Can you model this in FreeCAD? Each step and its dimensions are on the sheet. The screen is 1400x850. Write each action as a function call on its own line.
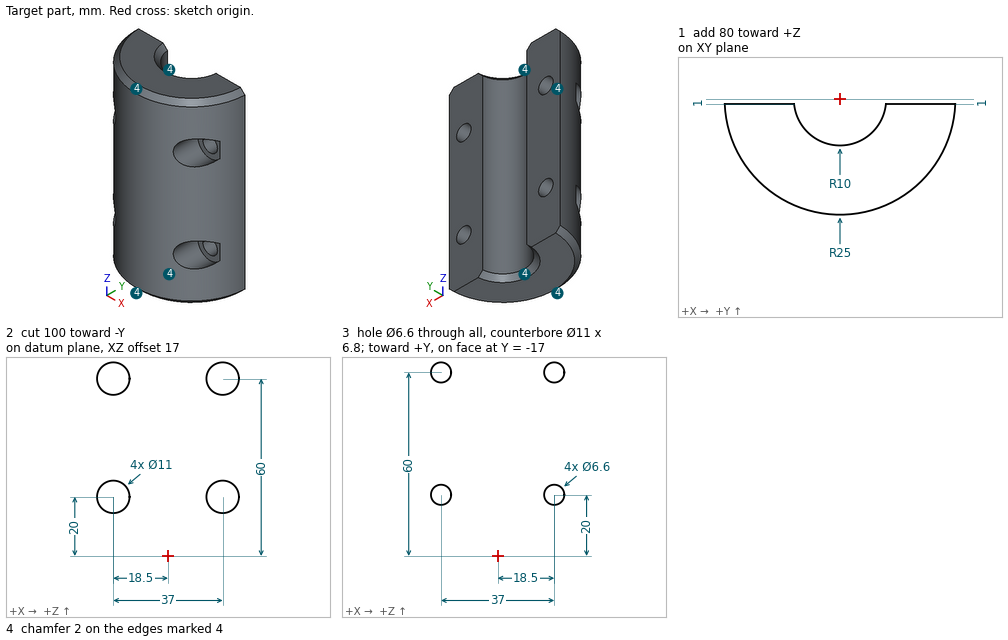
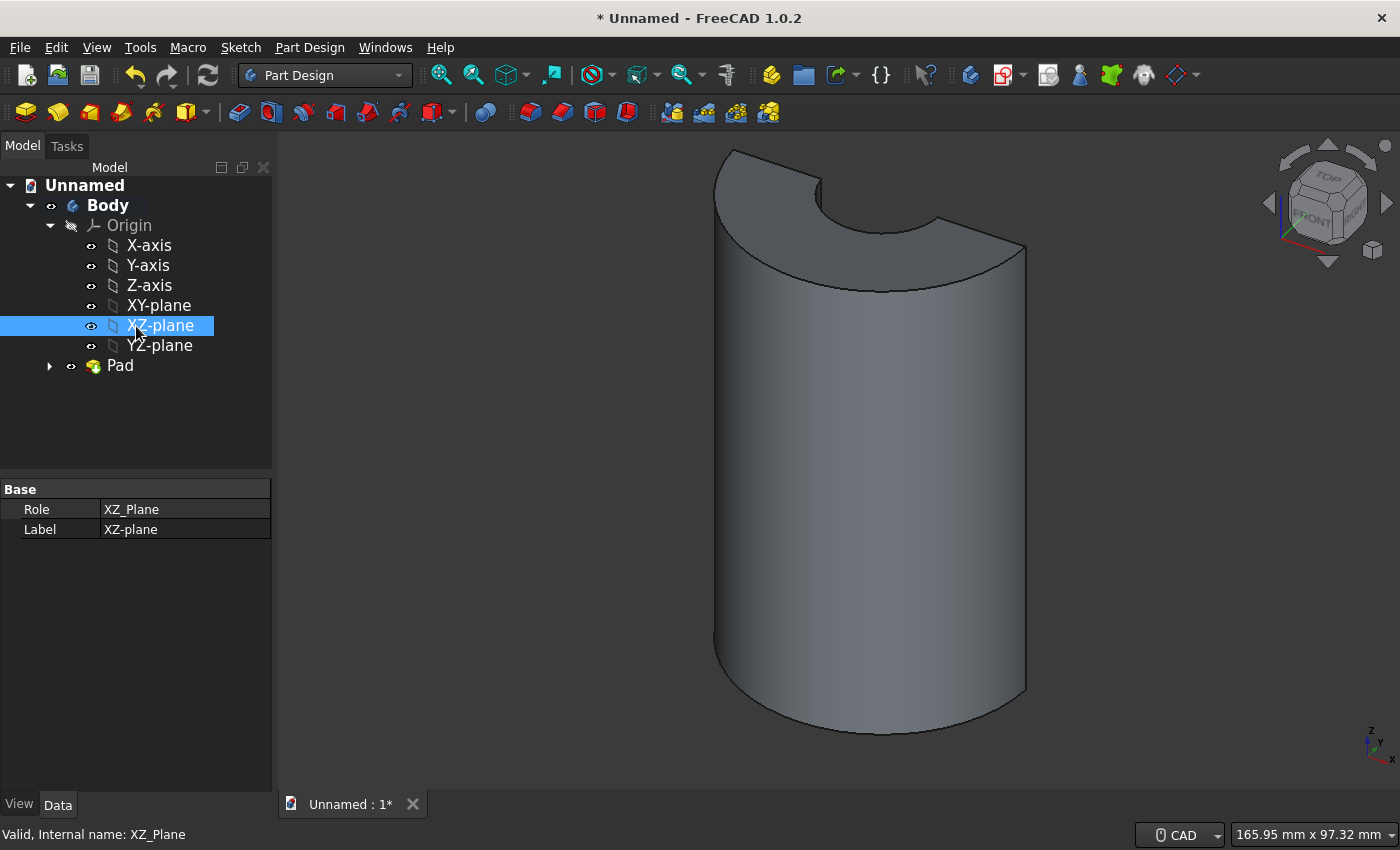
click(1176, 76)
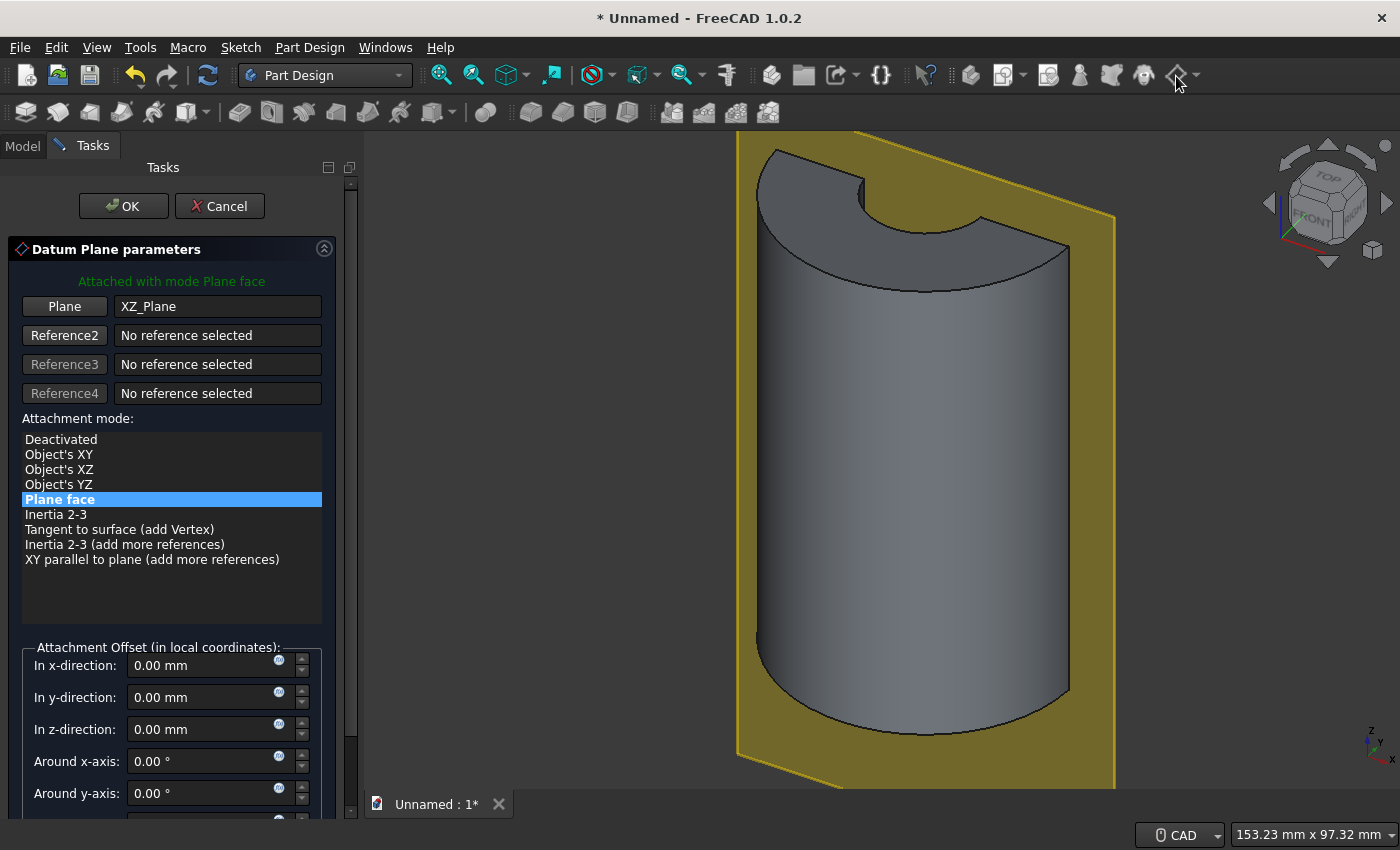
triple_click(210, 729)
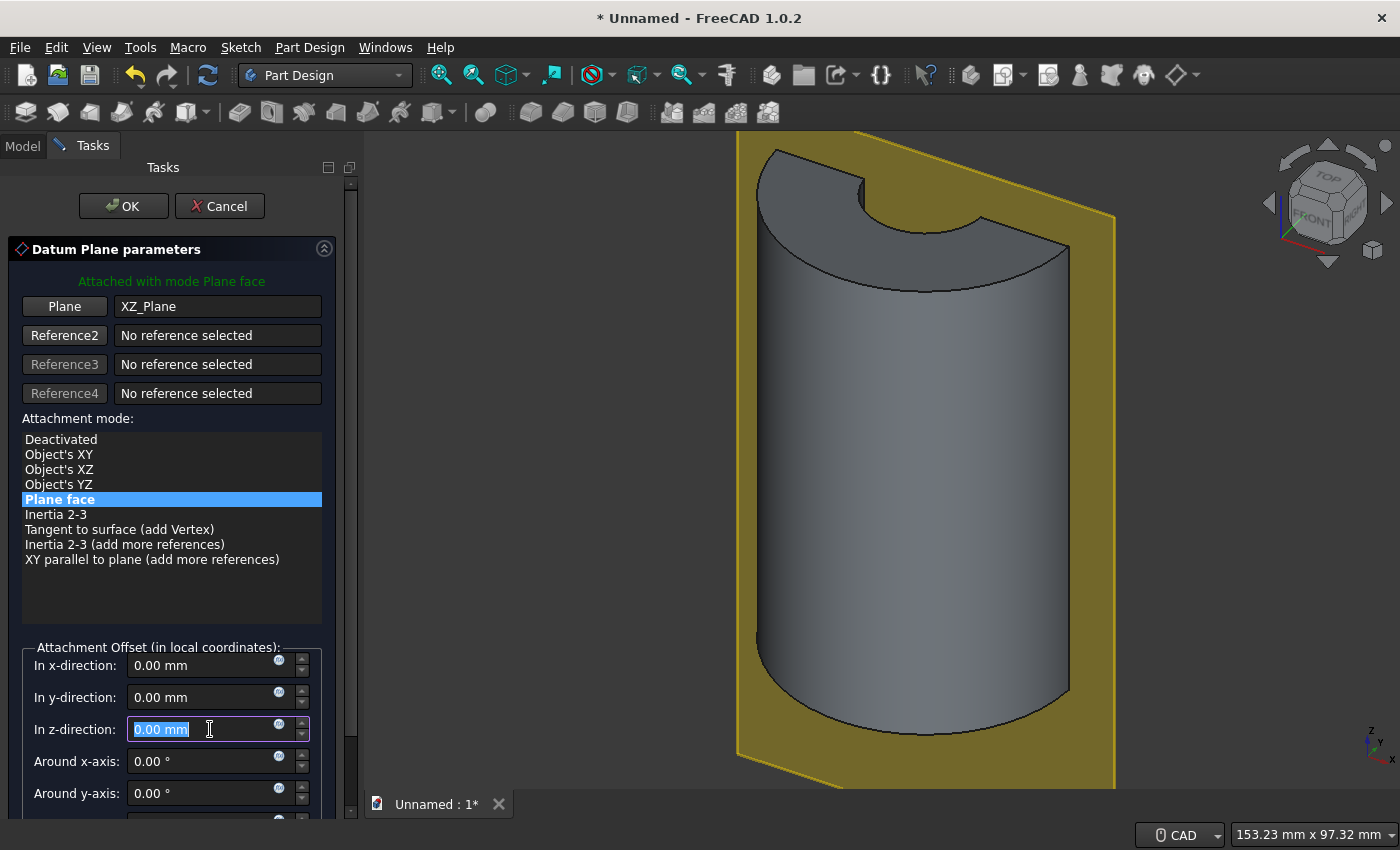
text(17)
key(Tab)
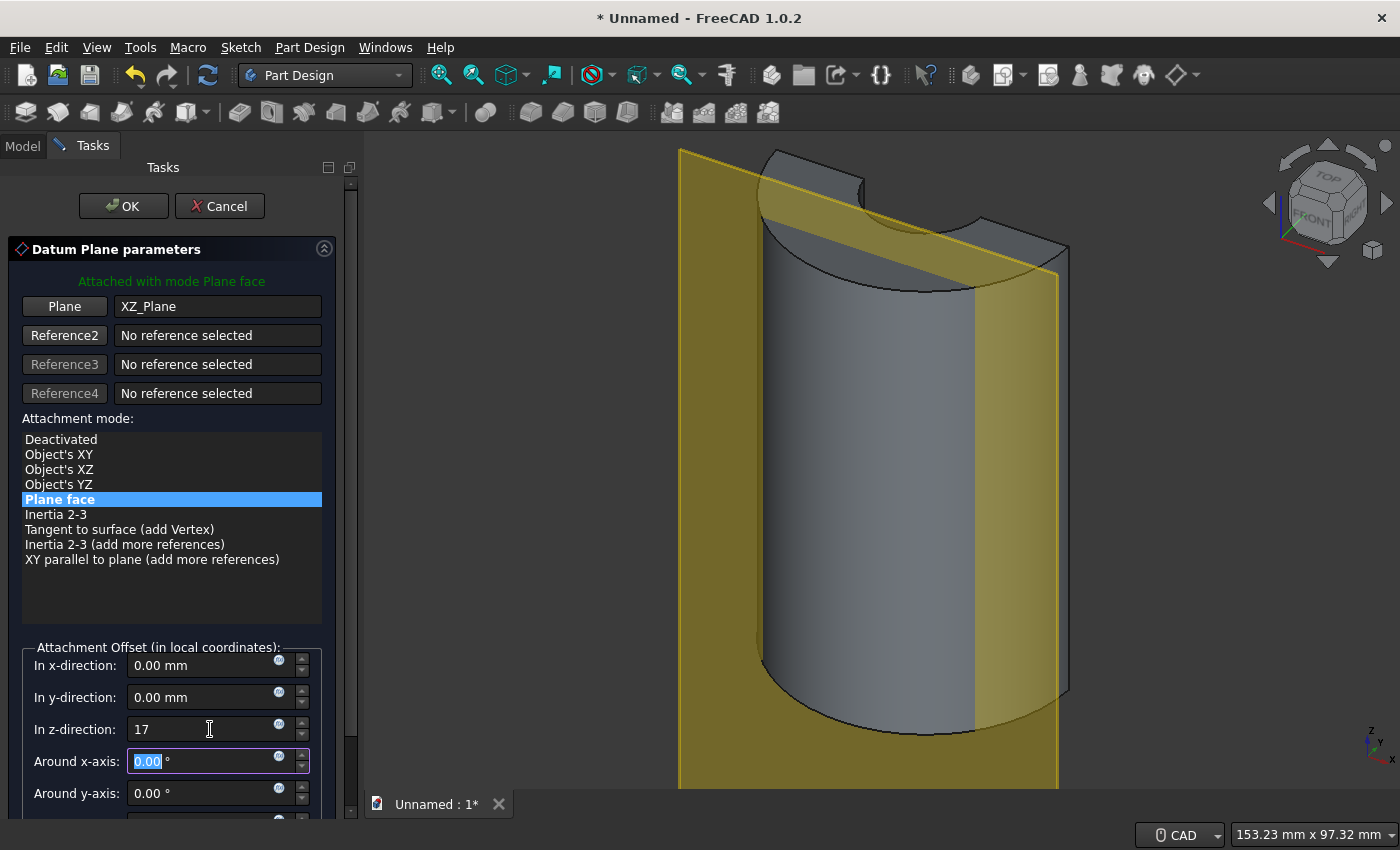
click(124, 206)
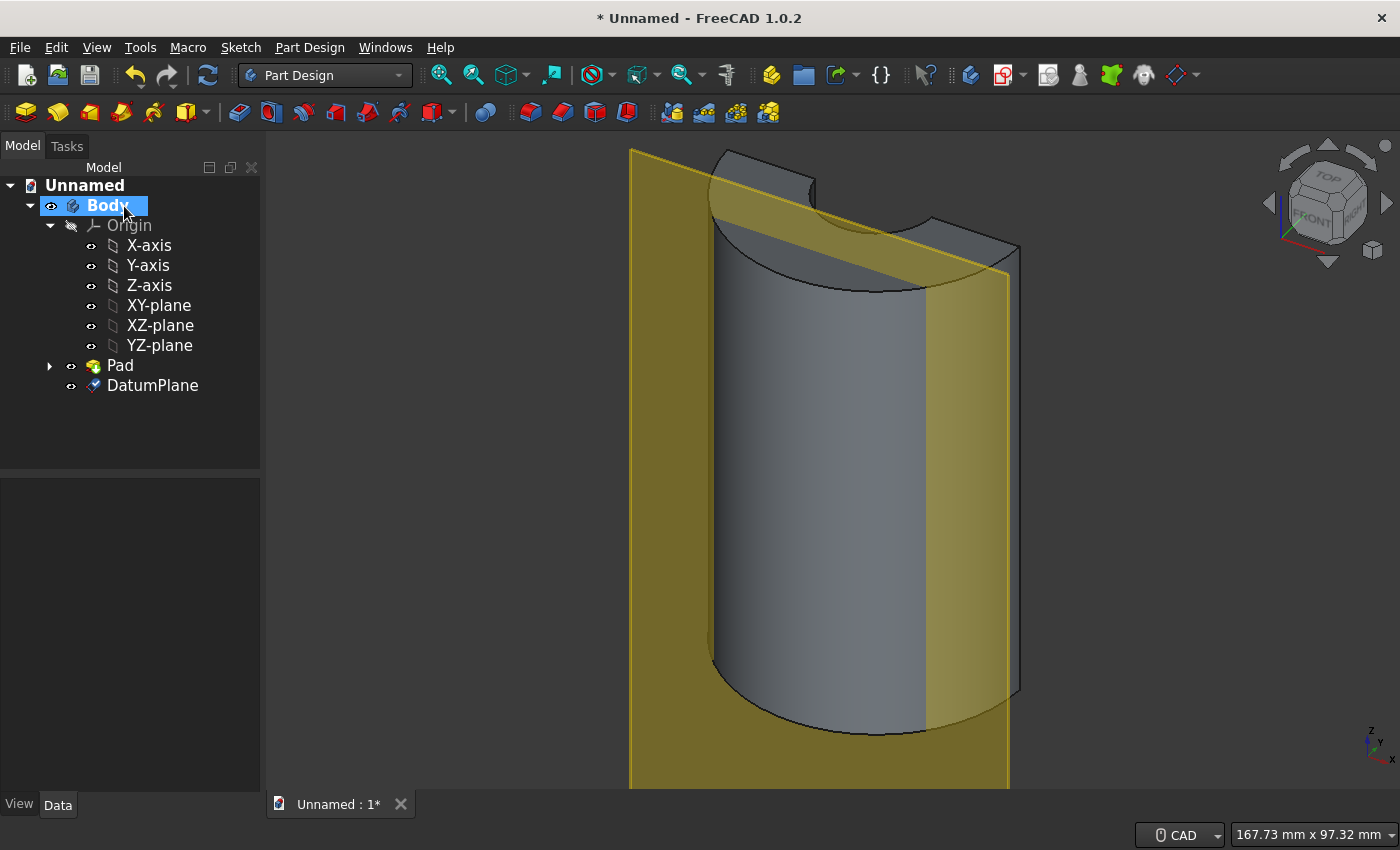
click(116, 386)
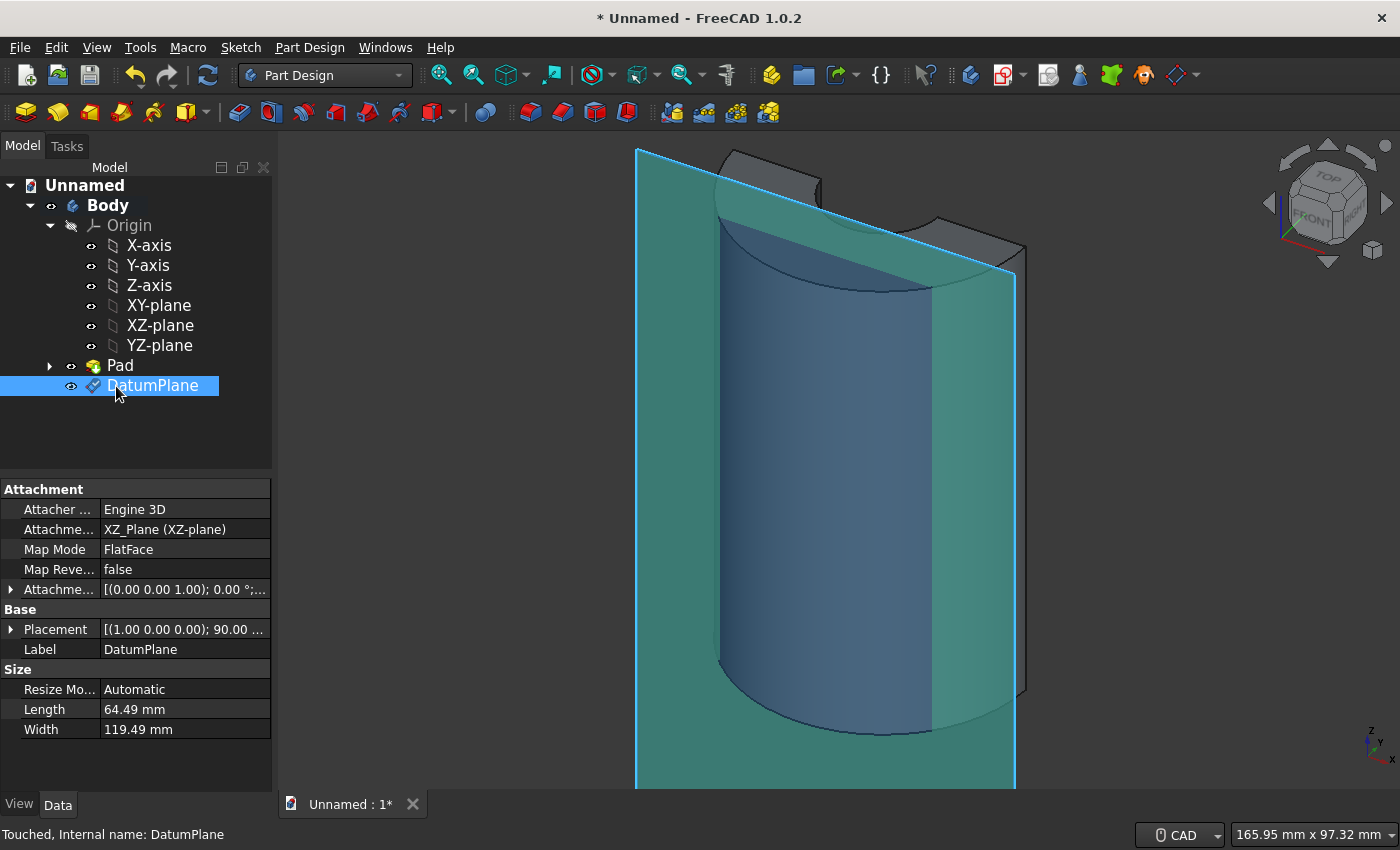
click(1004, 76)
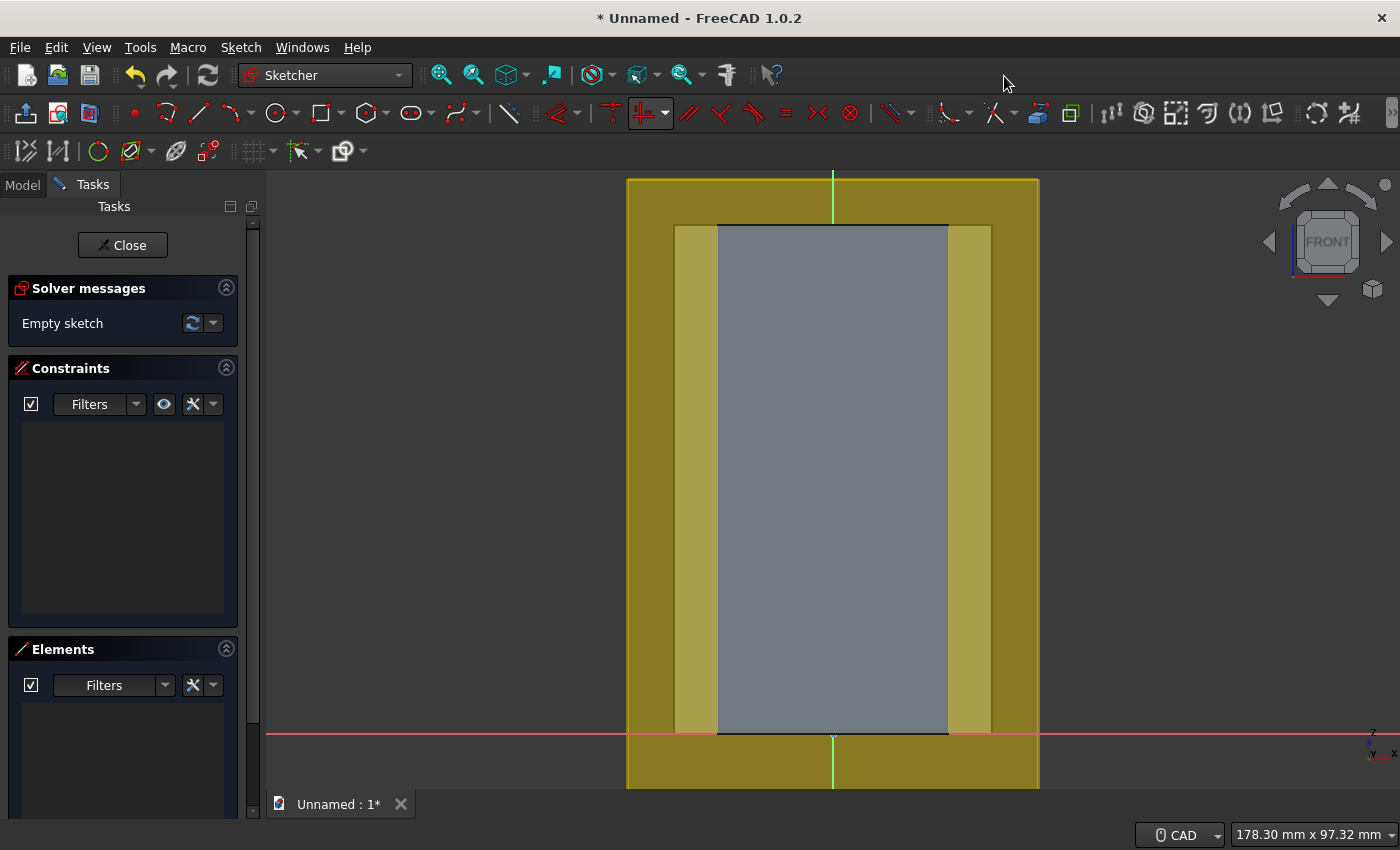
click(90, 114)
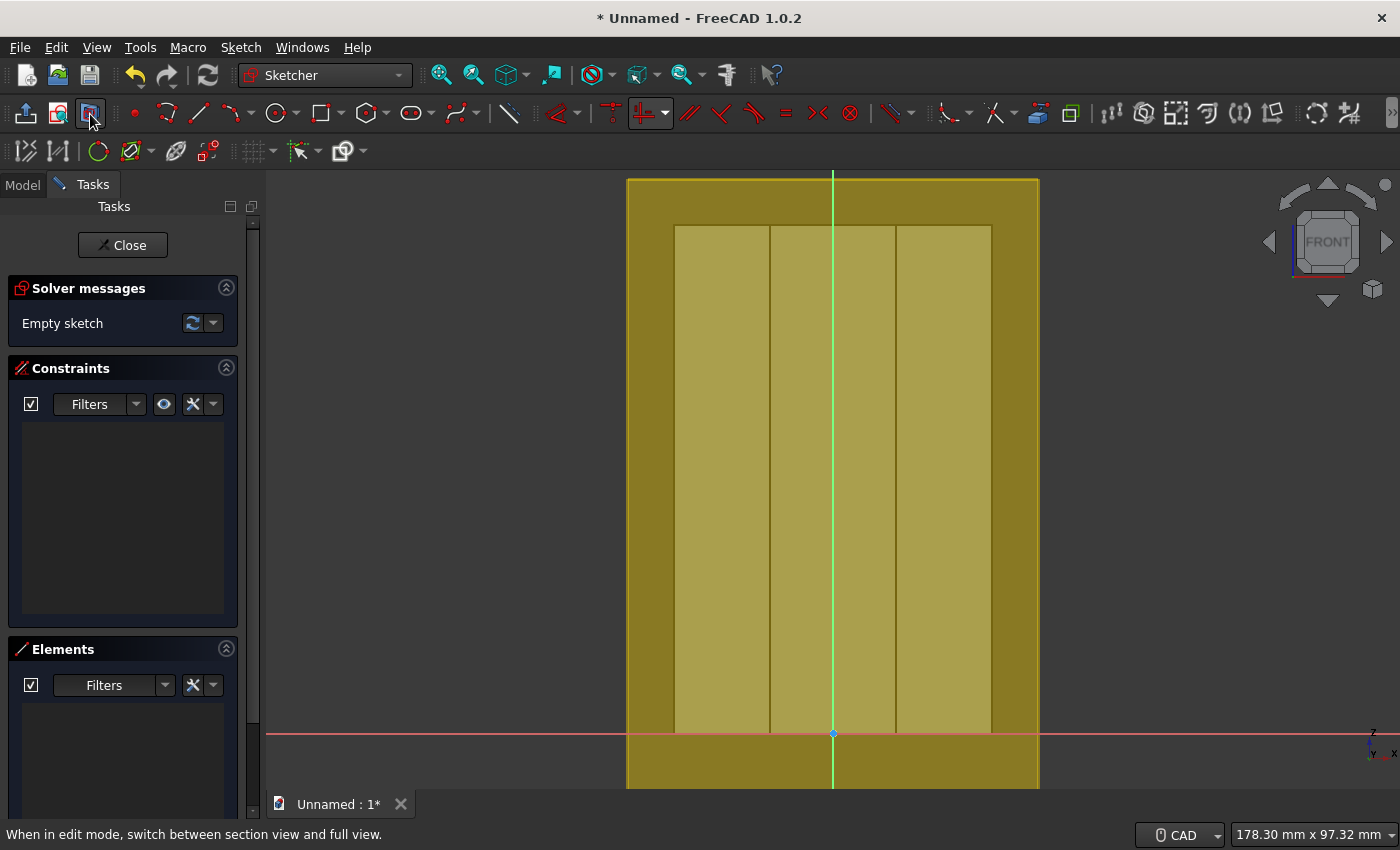
click(276, 114)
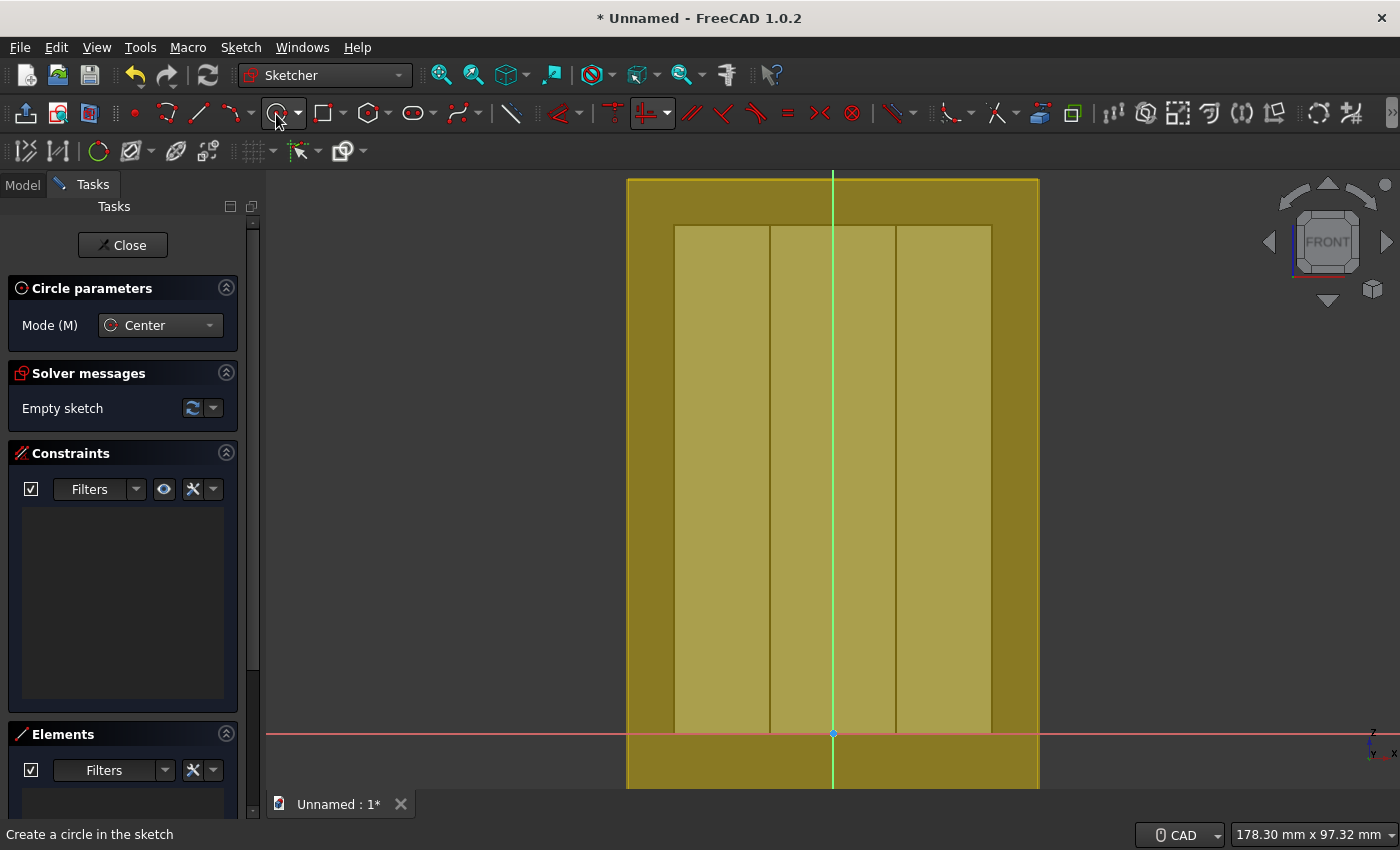
click(715, 607)
move(740, 582)